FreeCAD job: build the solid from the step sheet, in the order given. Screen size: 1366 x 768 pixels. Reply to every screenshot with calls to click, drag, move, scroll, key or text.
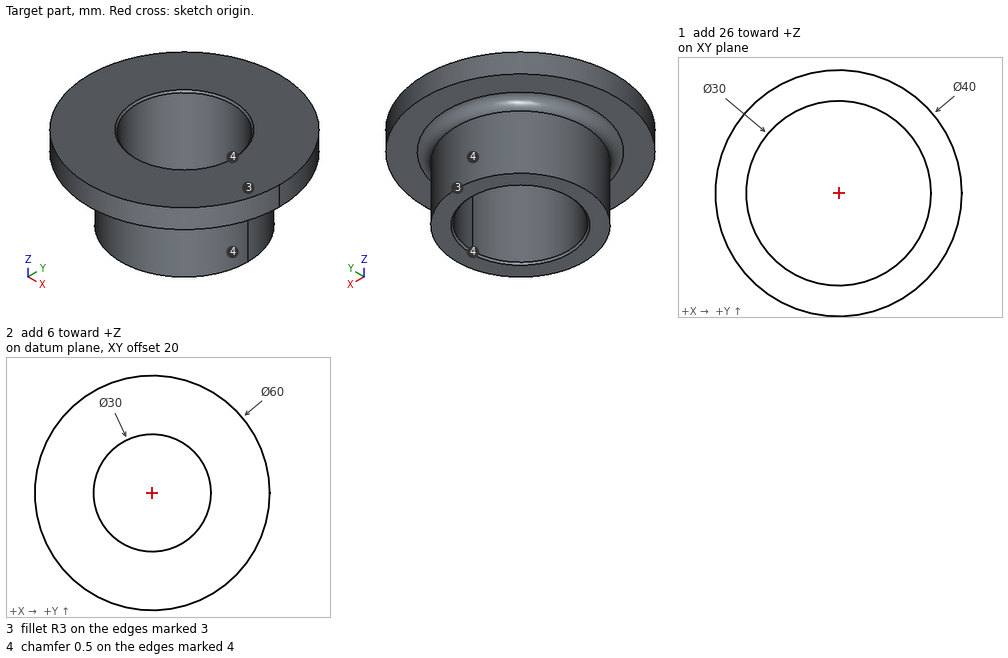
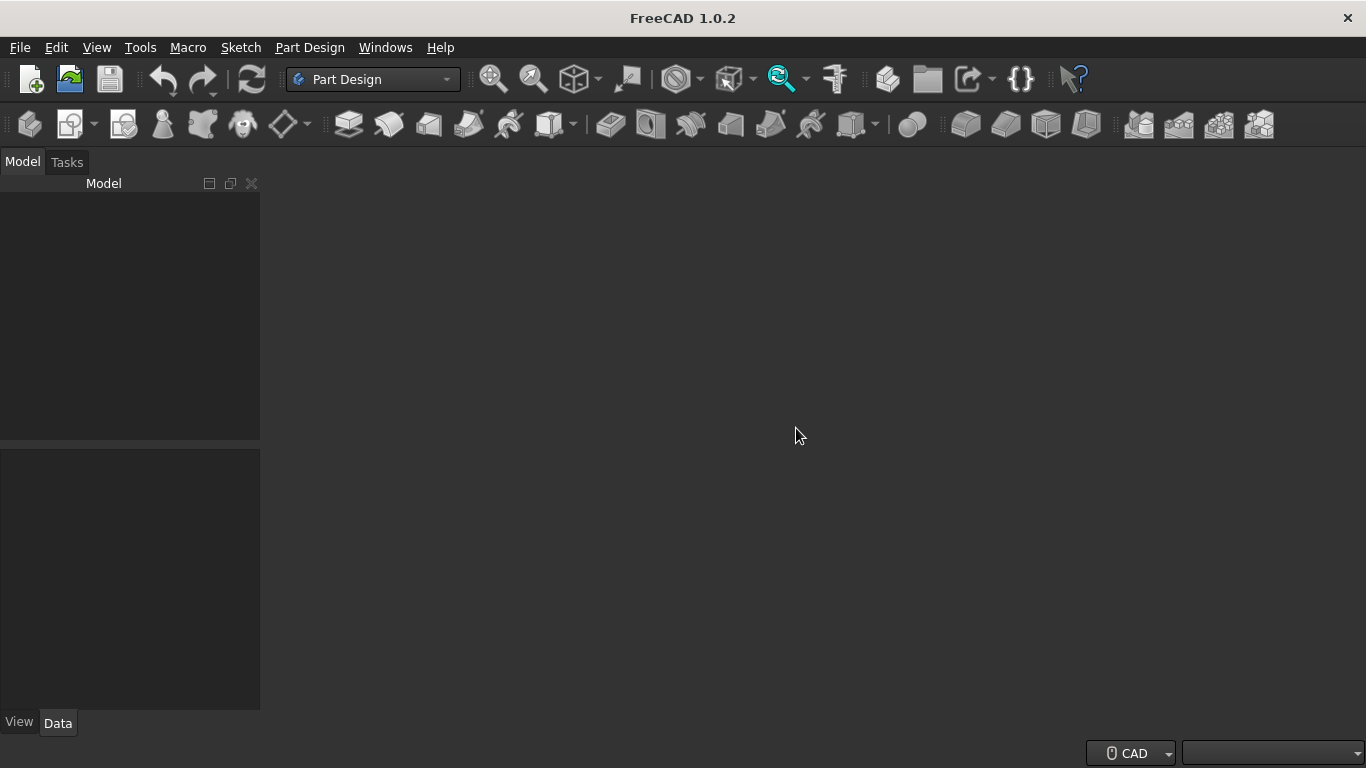
key(ctrl+n)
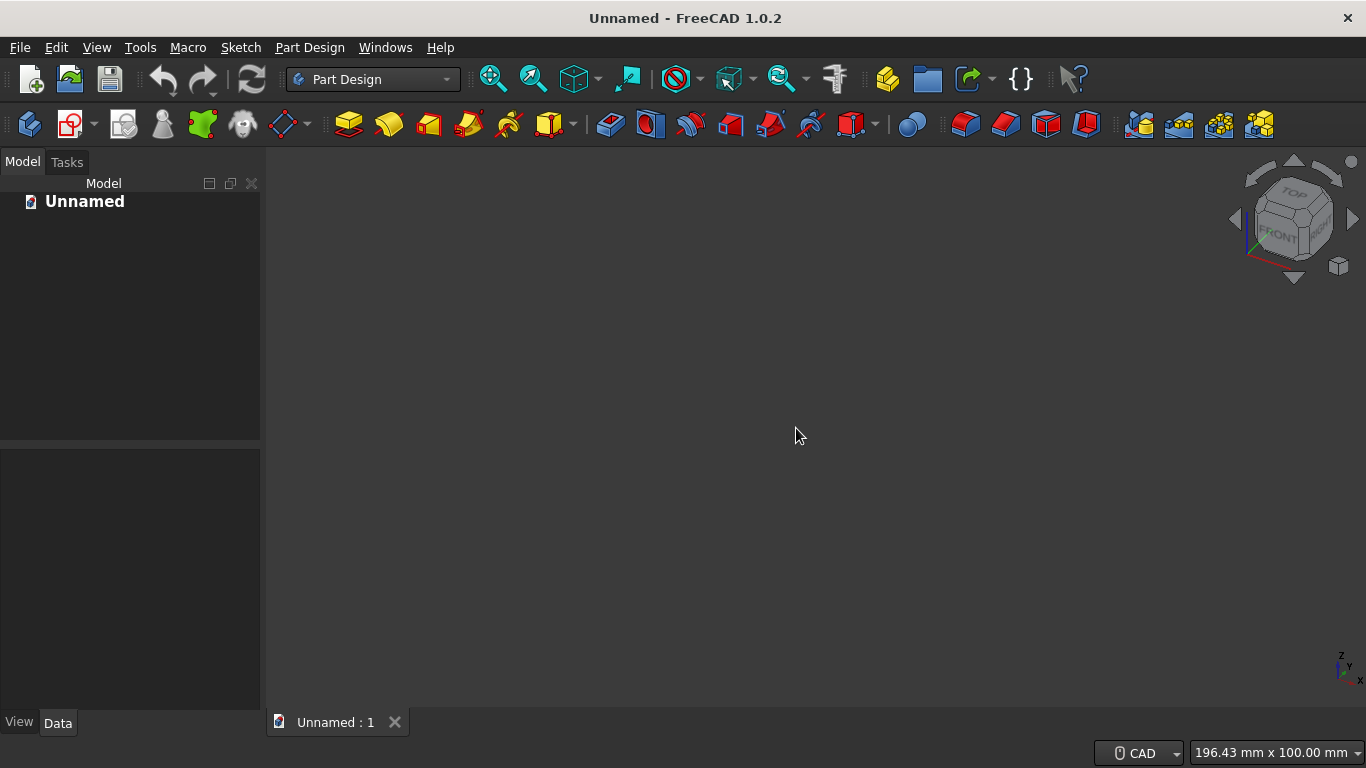
click(70, 124)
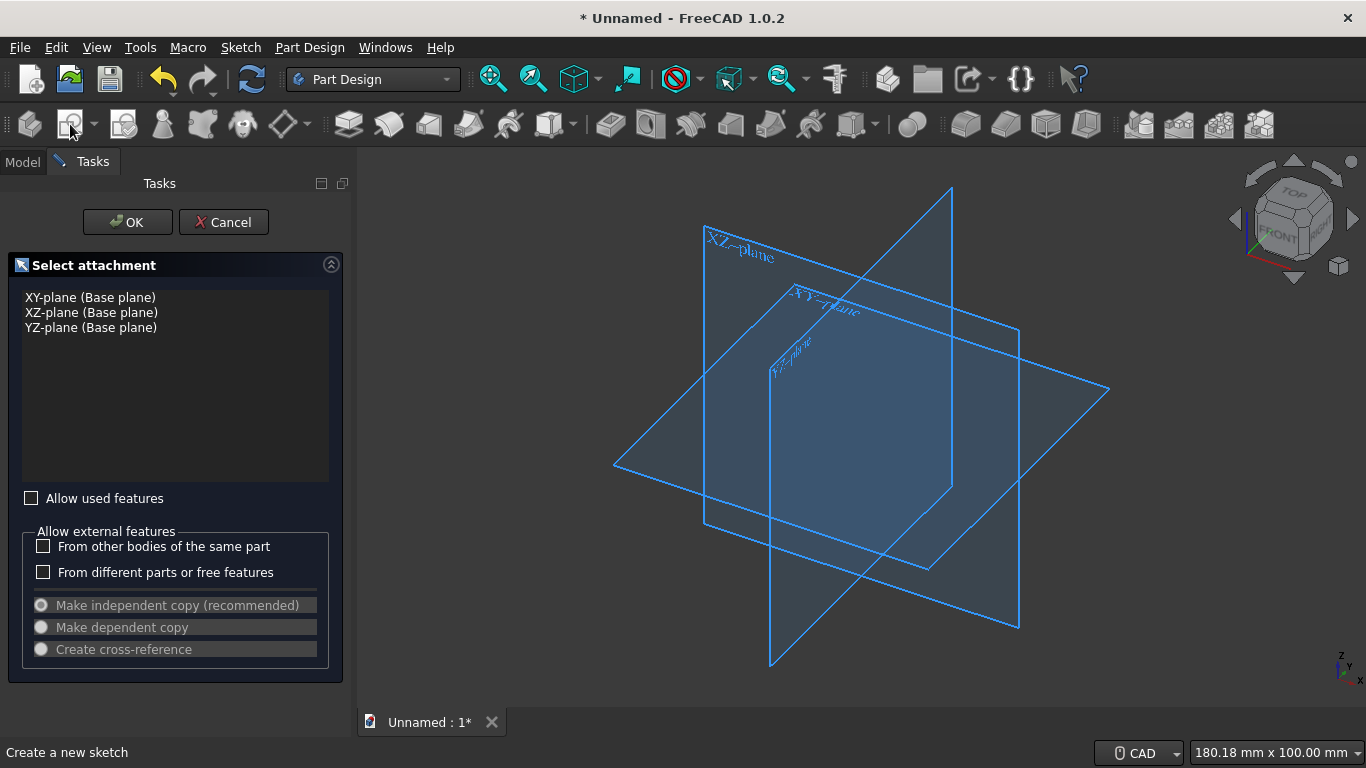
click(82, 298)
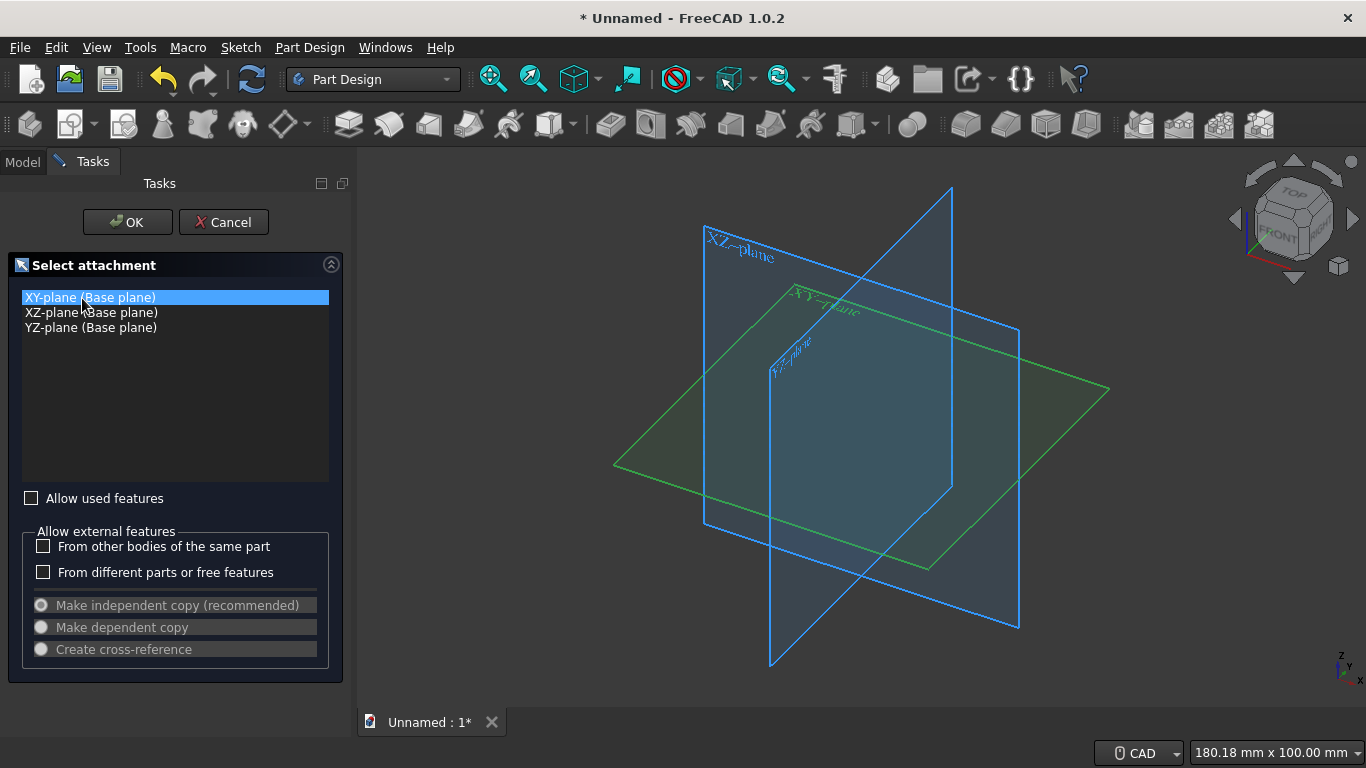
click(128, 222)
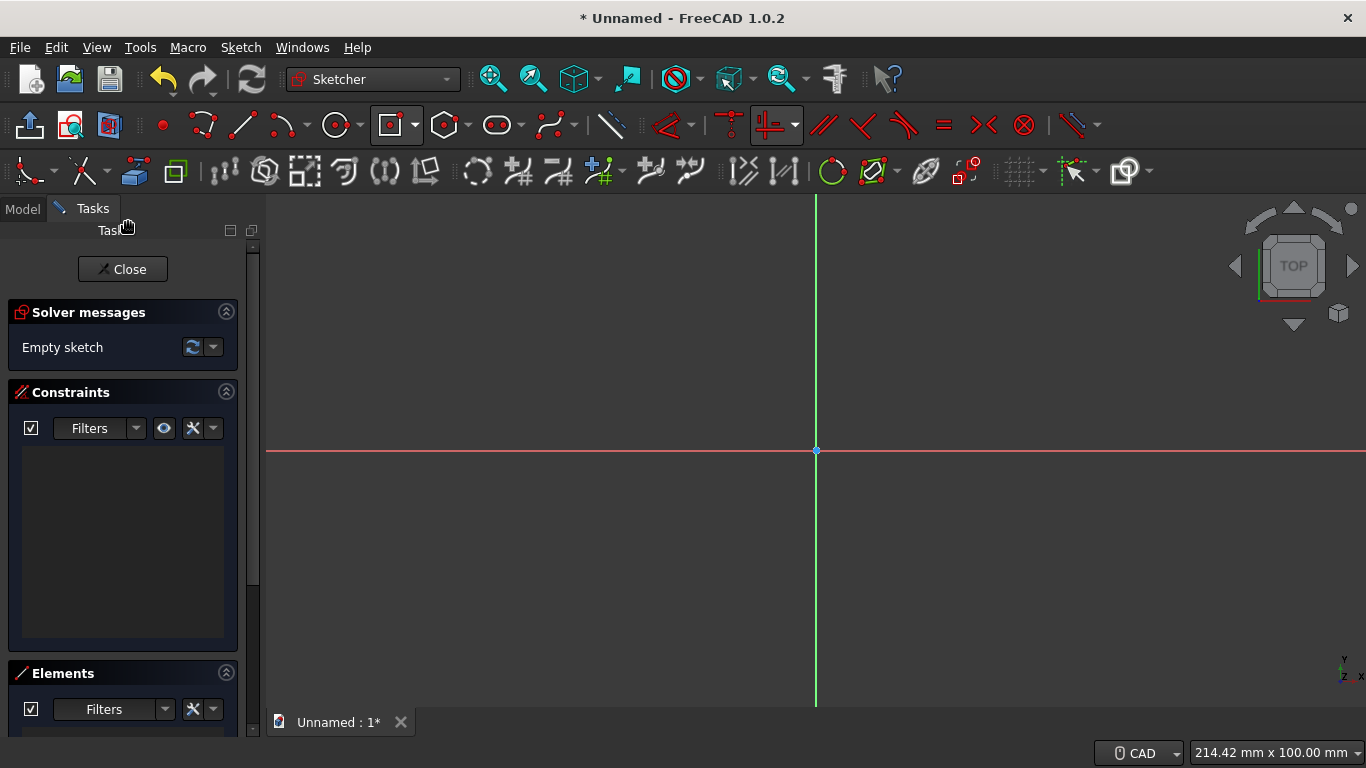
scroll(955, 451, up, 2)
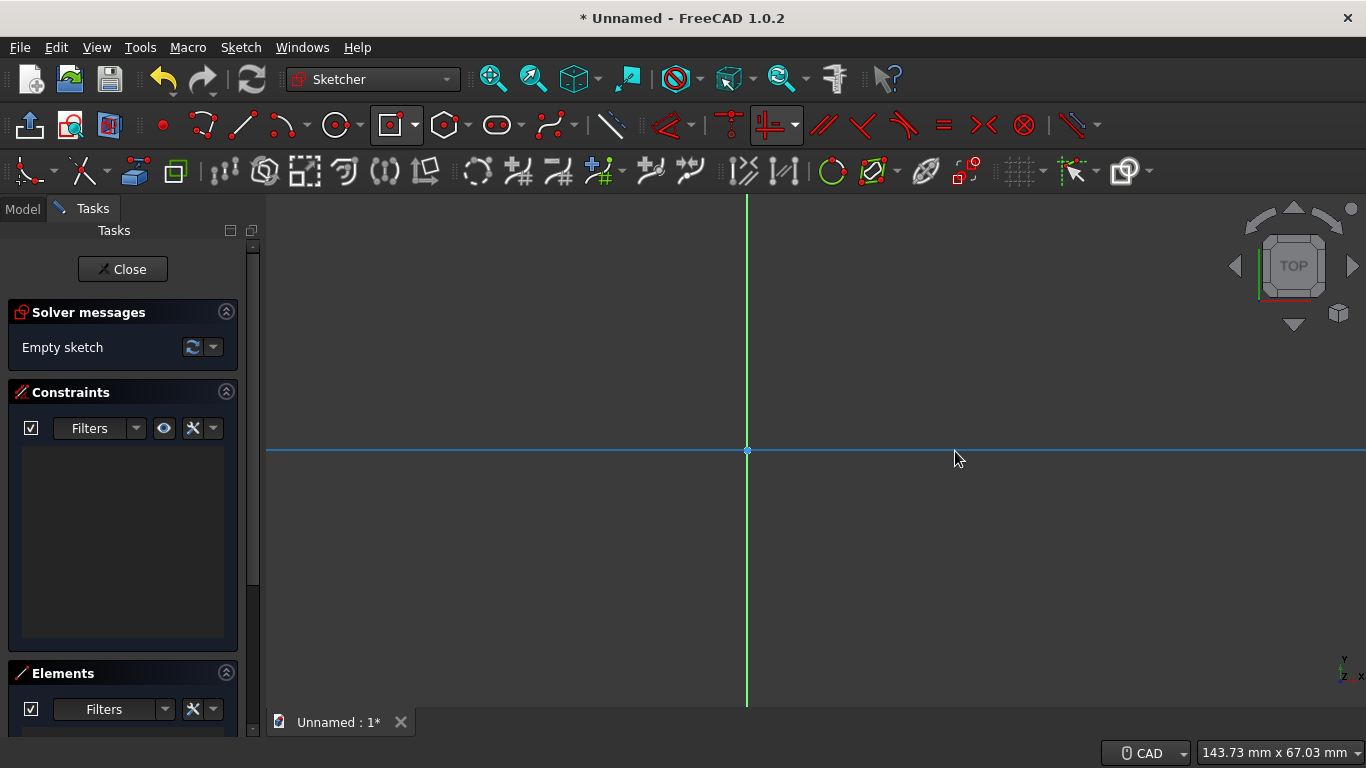
click(336, 126)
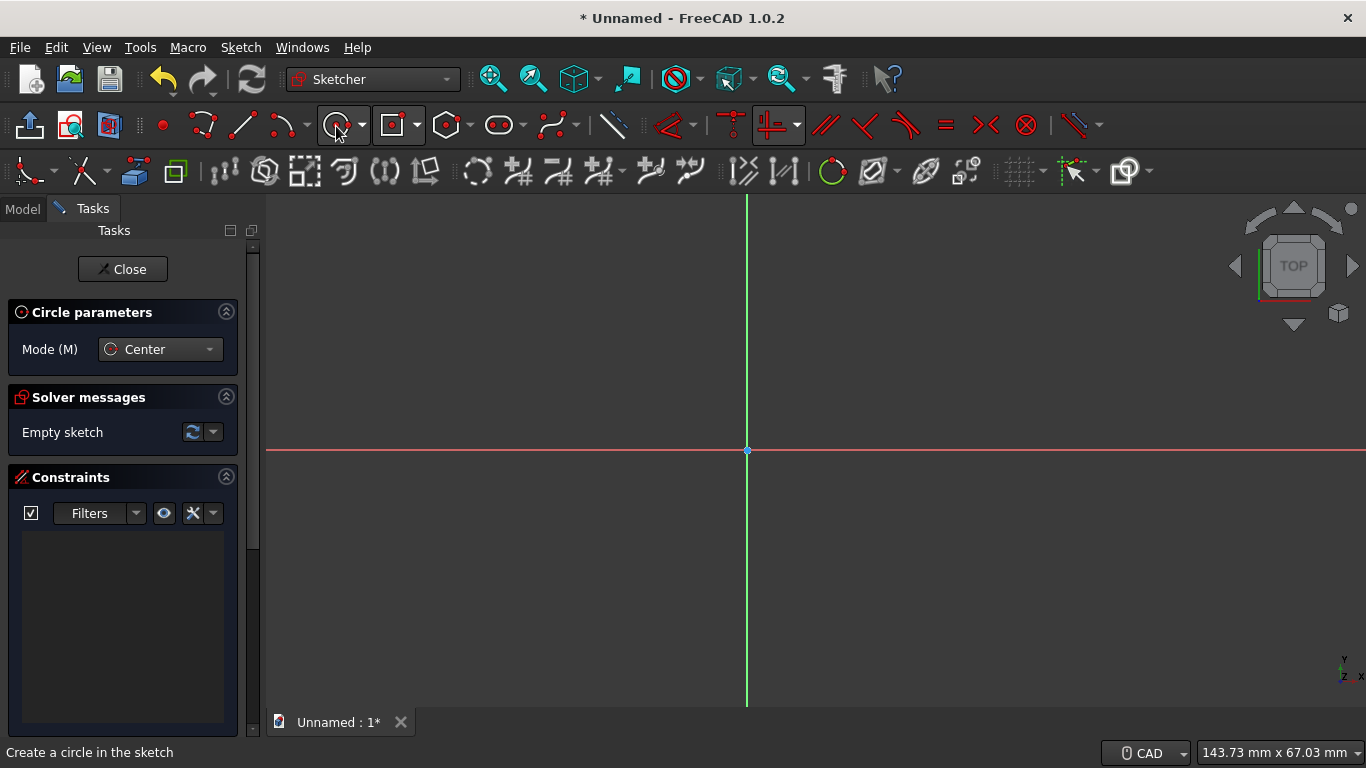
click(747, 450)
move(856, 342)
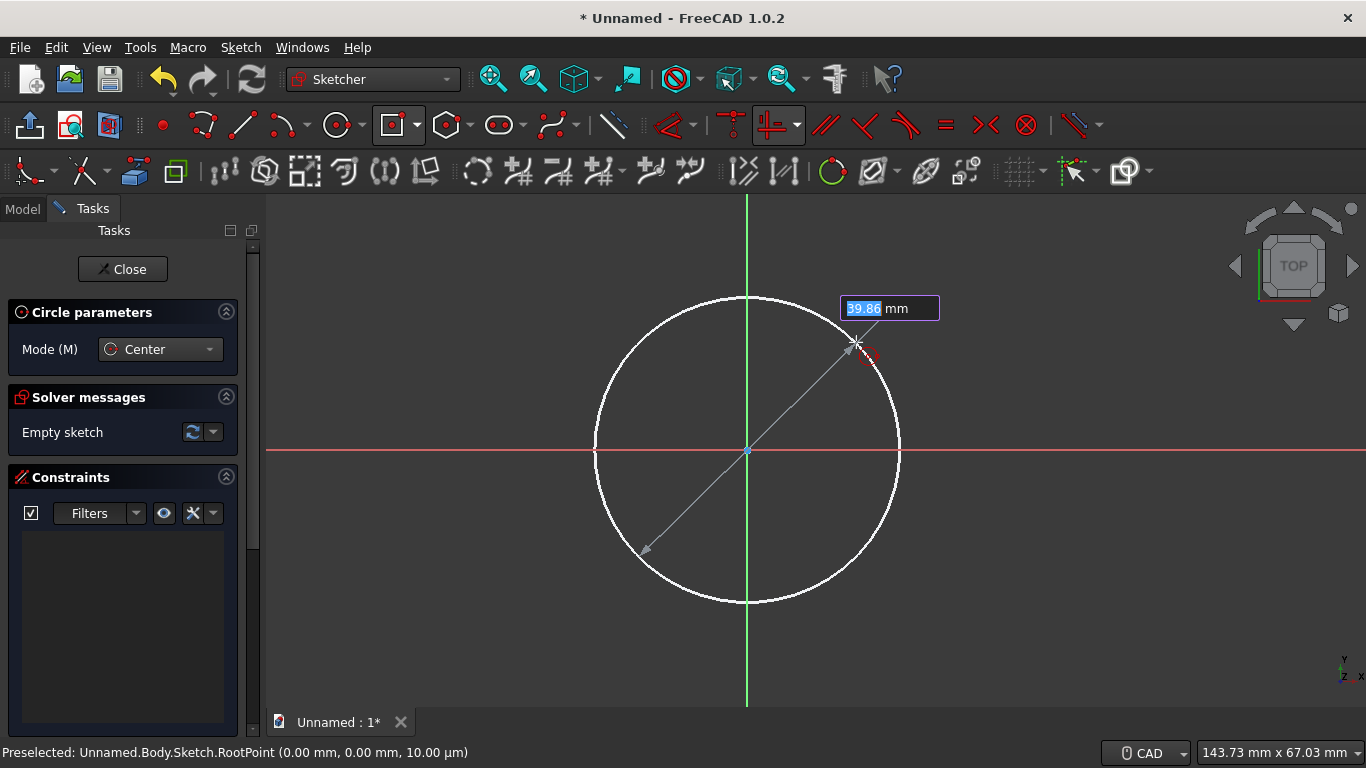
text(40)
key(Return)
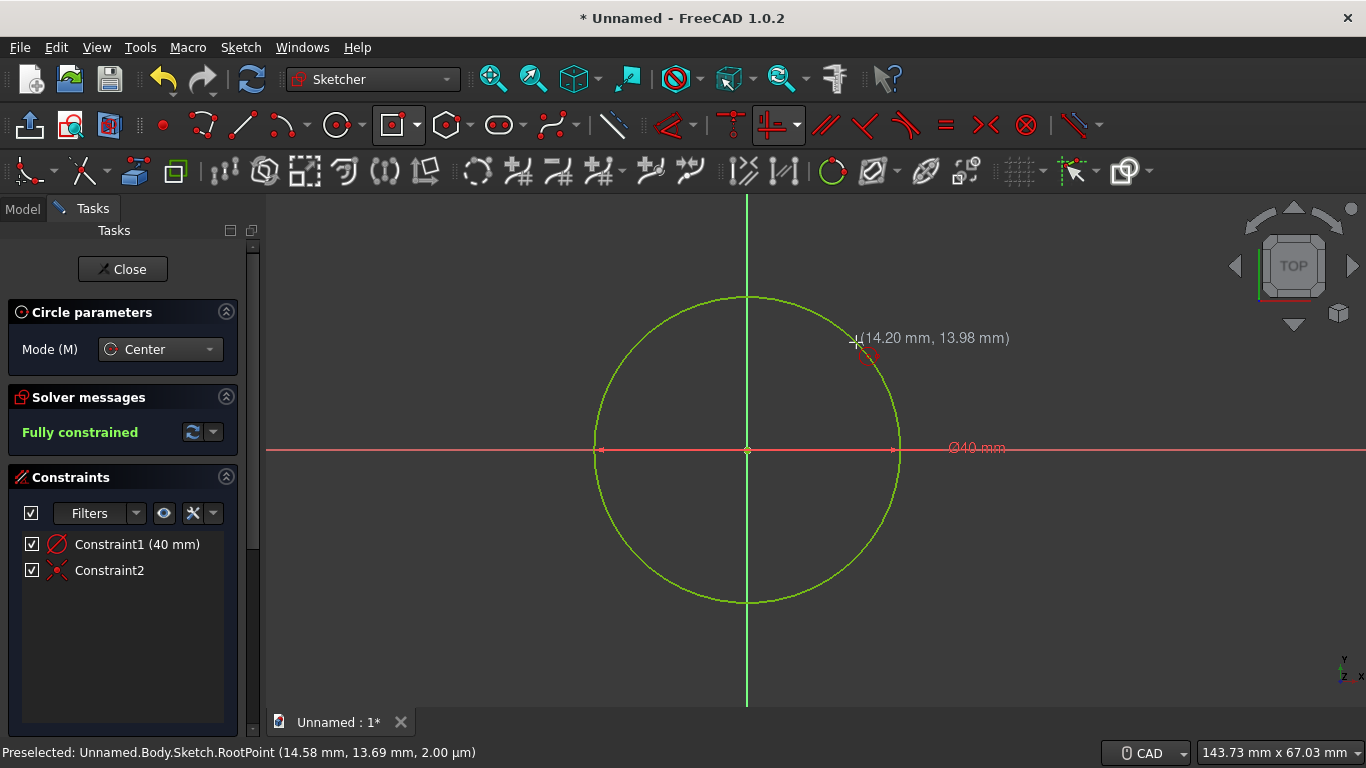
click(747, 450)
move(829, 369)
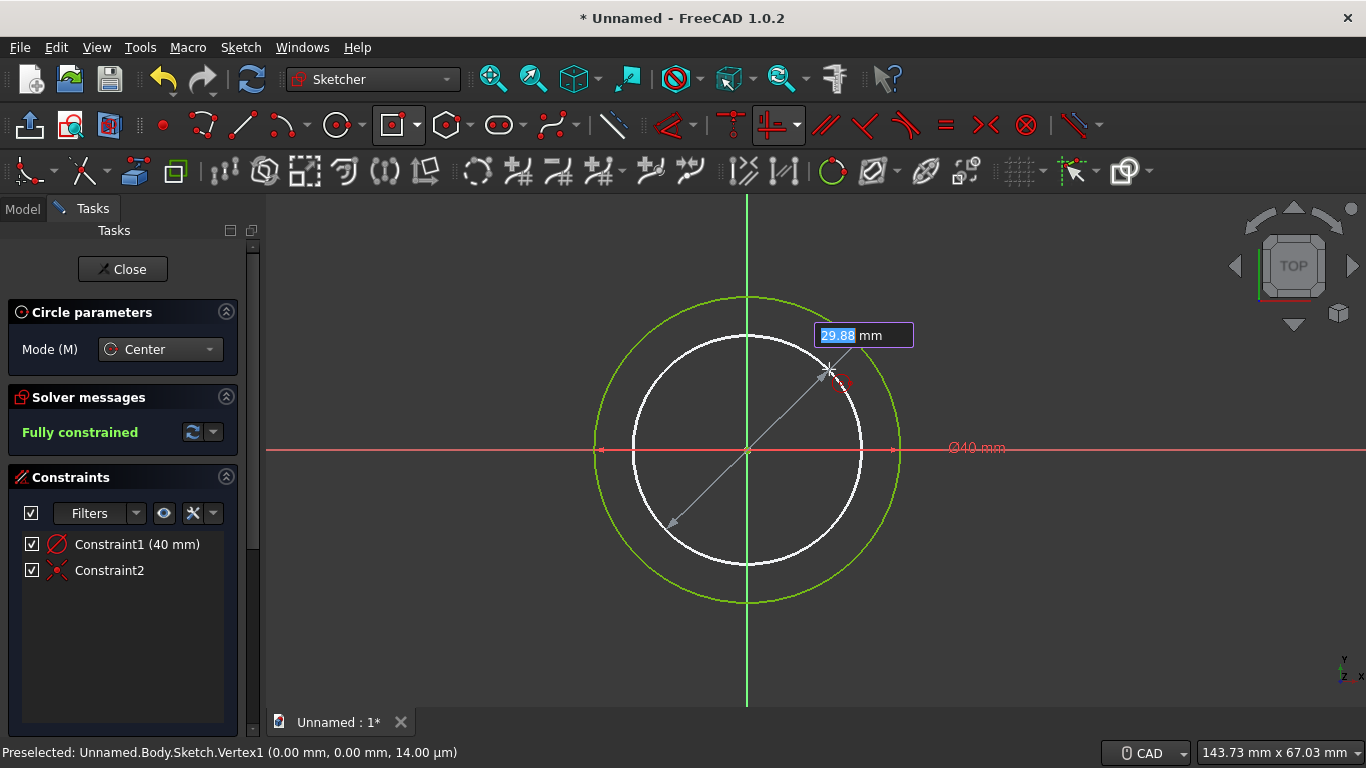
text(30)
key(Return)
key(Escape)